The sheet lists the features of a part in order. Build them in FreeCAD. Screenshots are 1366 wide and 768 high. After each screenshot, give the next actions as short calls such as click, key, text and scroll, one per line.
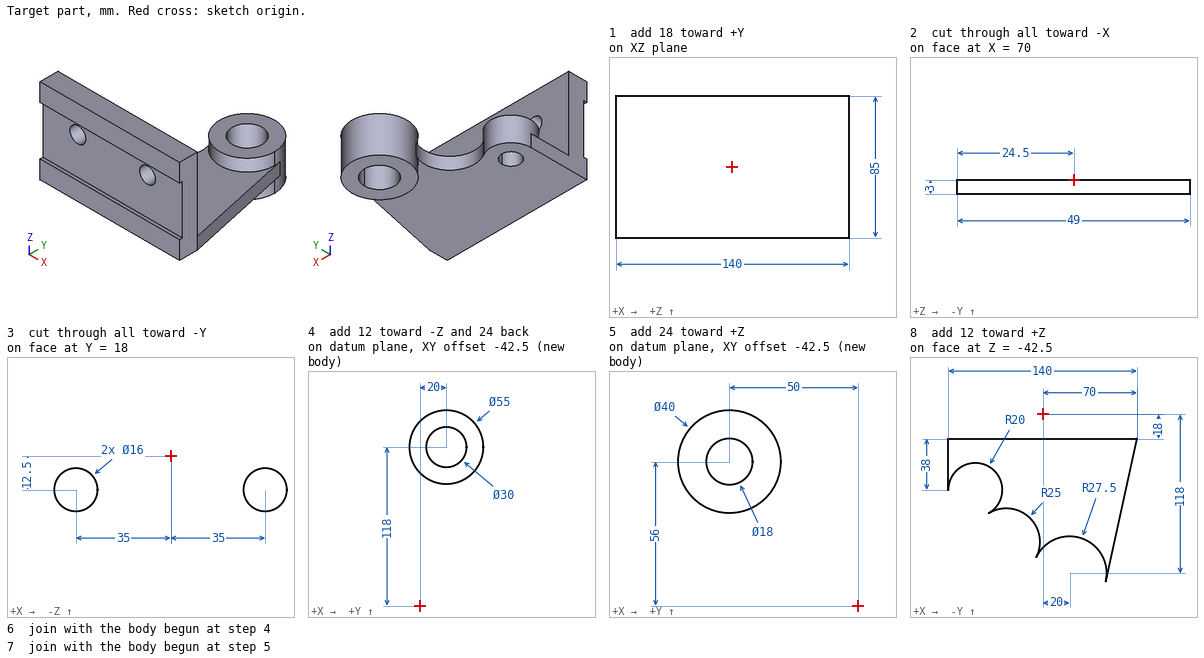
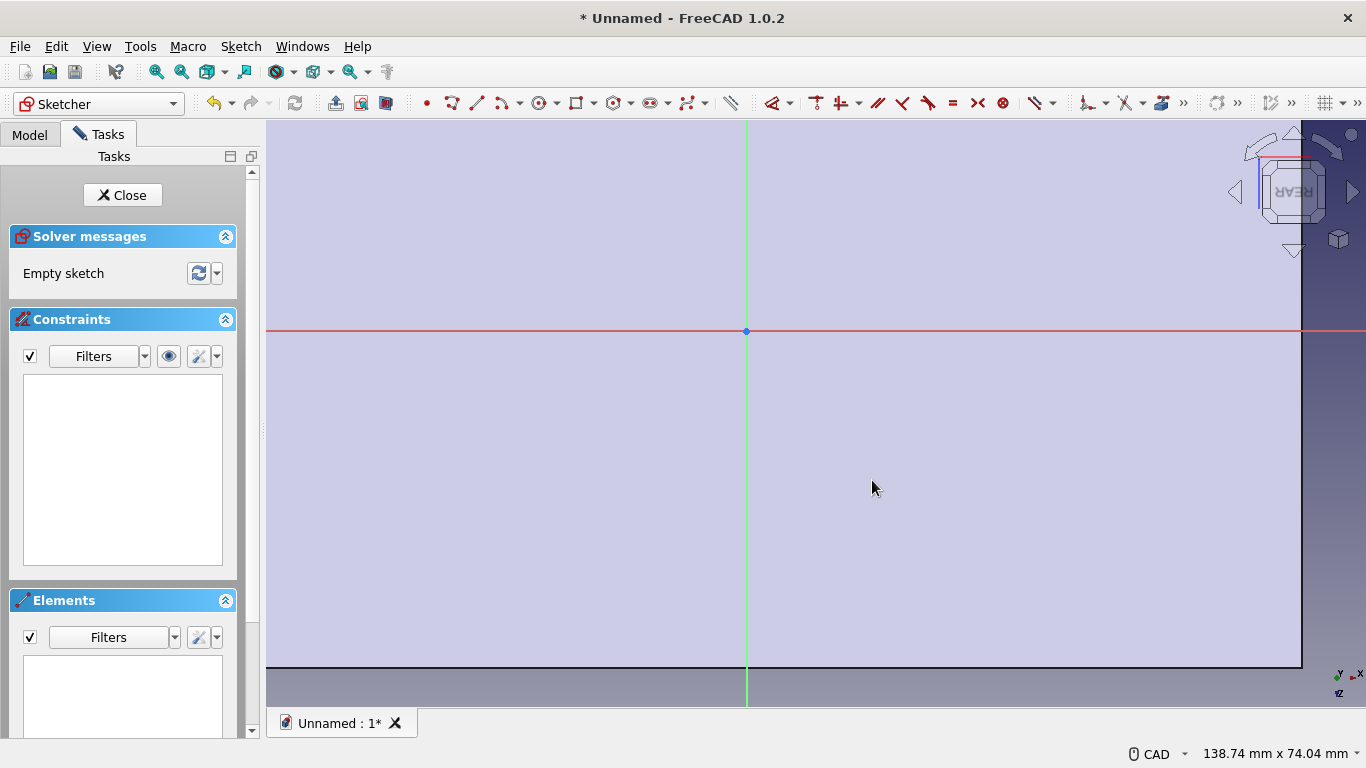
click(538, 104)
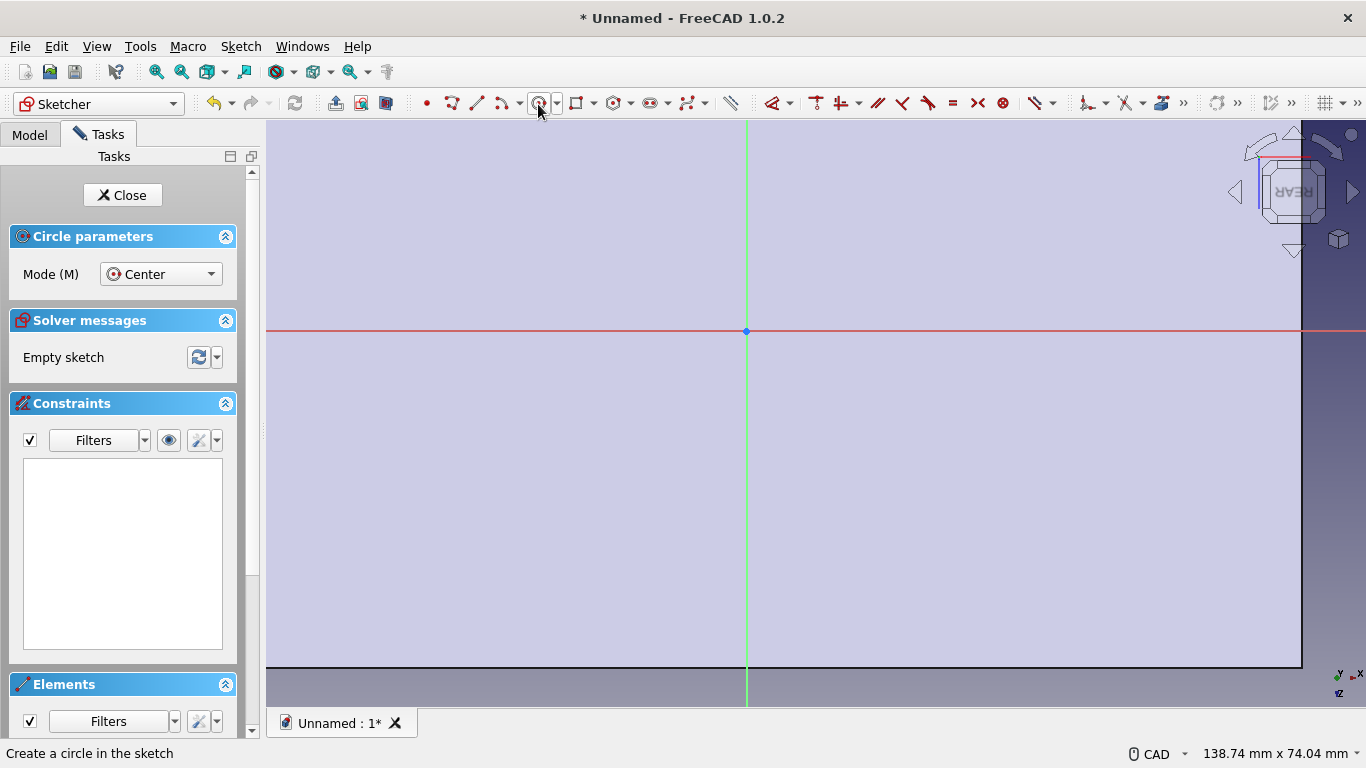
click(469, 430)
click(514, 386)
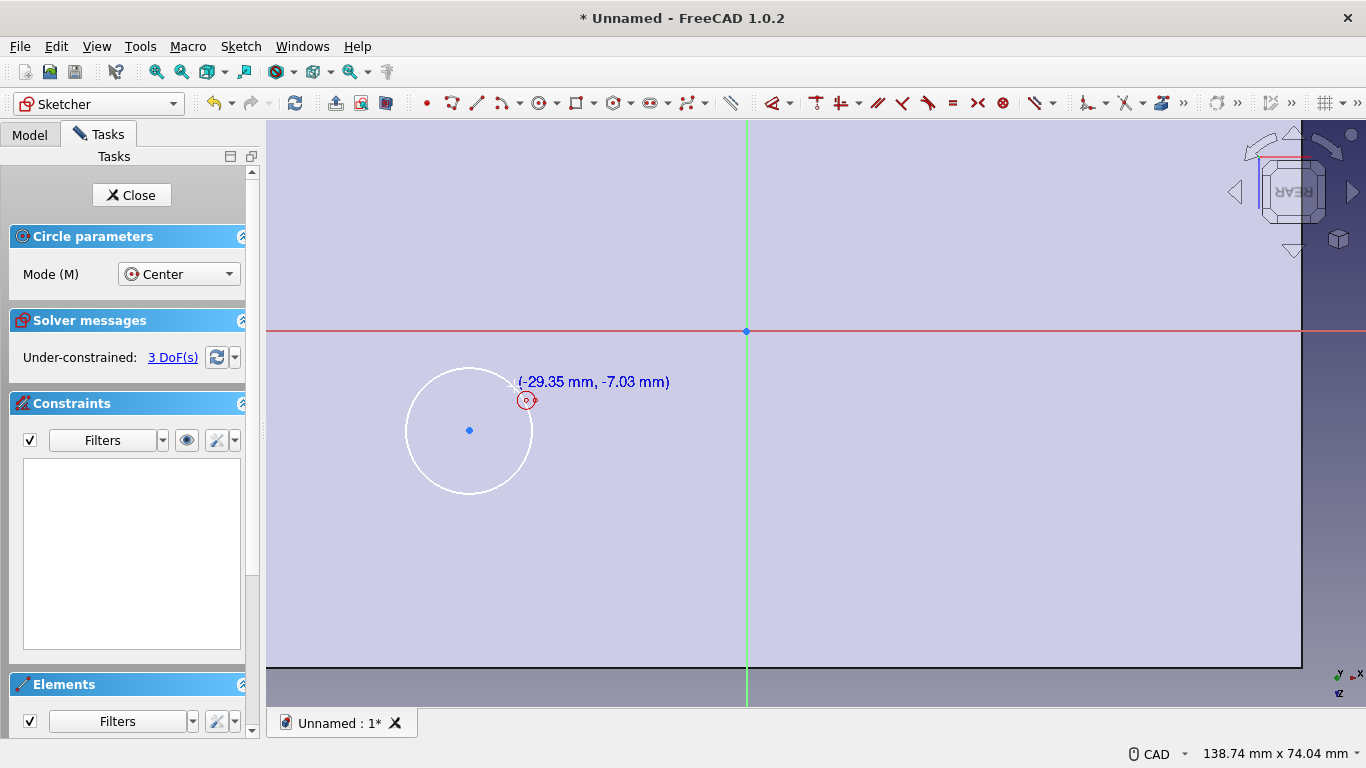
click(1024, 430)
click(1069, 386)
key(Escape)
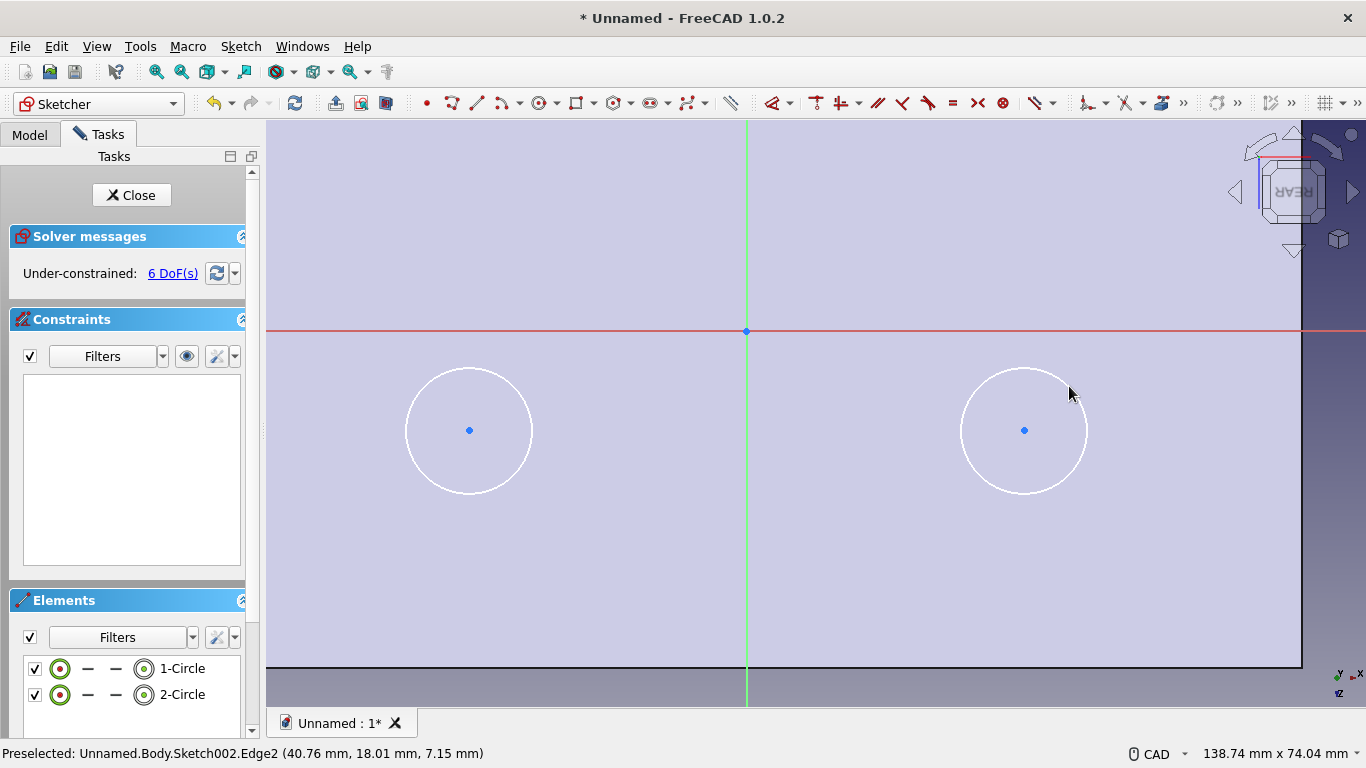
click(513, 386)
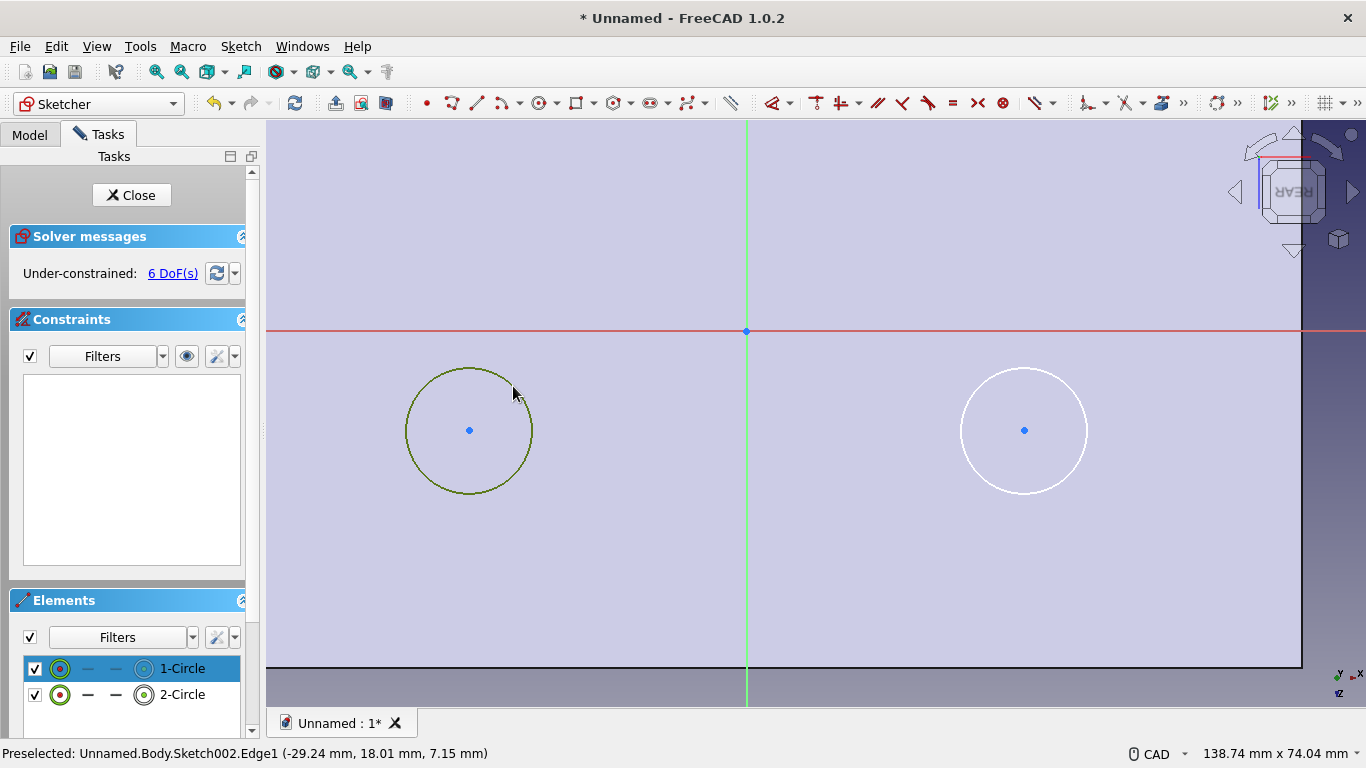
click(1068, 386)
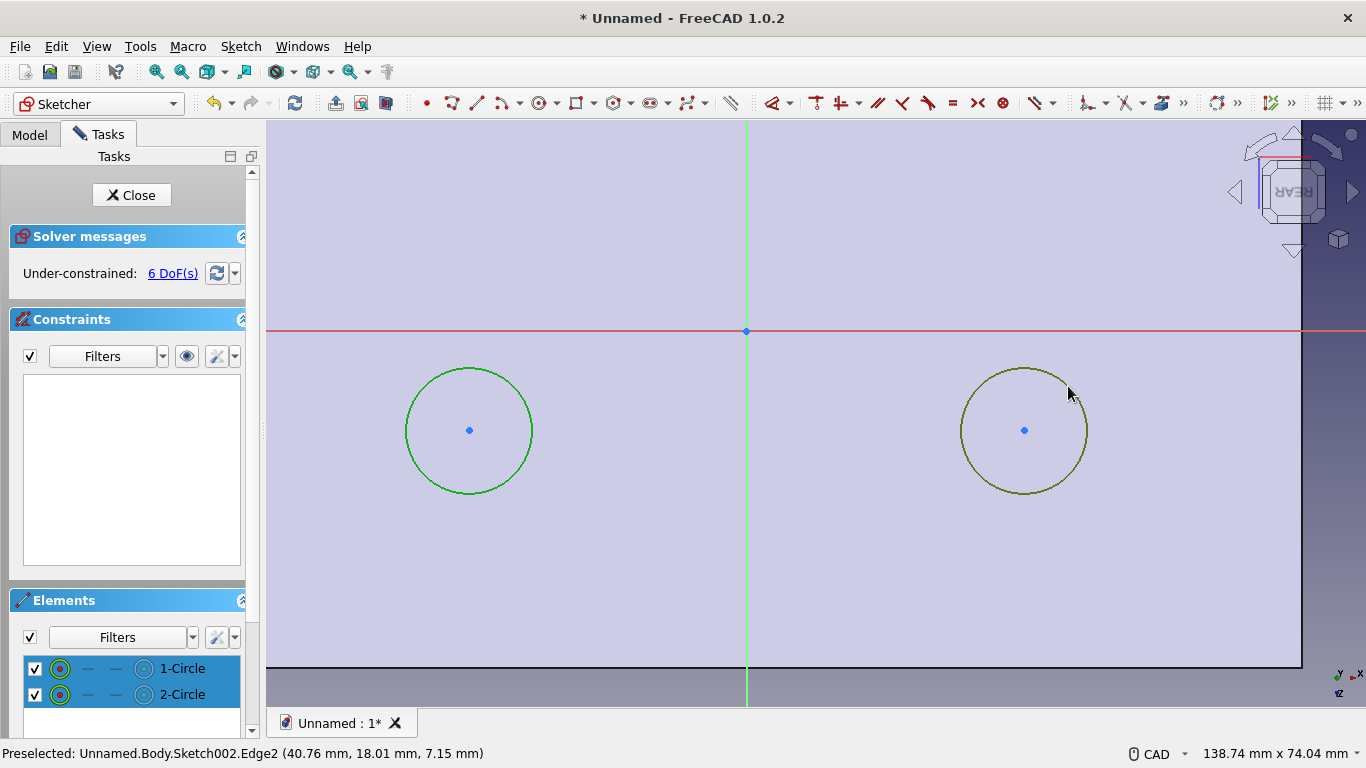
click(953, 104)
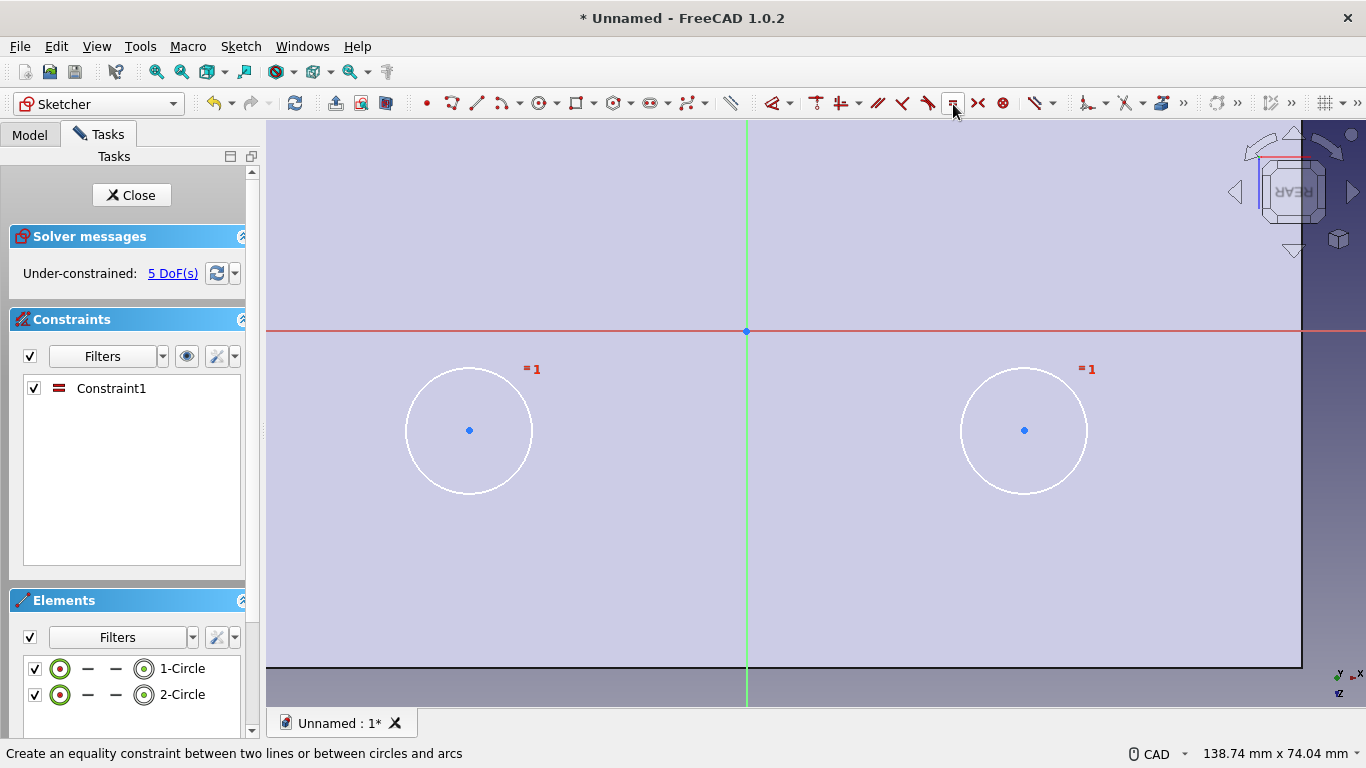
click(469, 431)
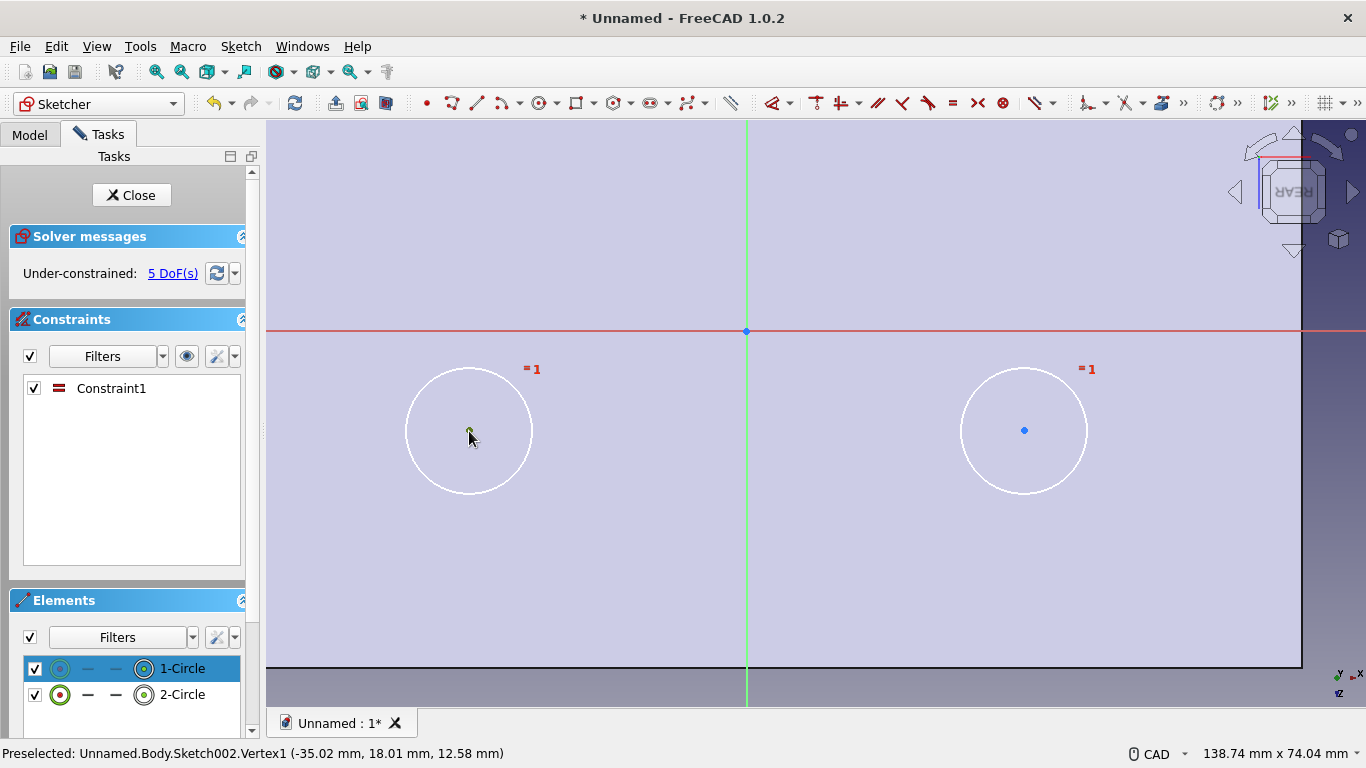
click(1024, 431)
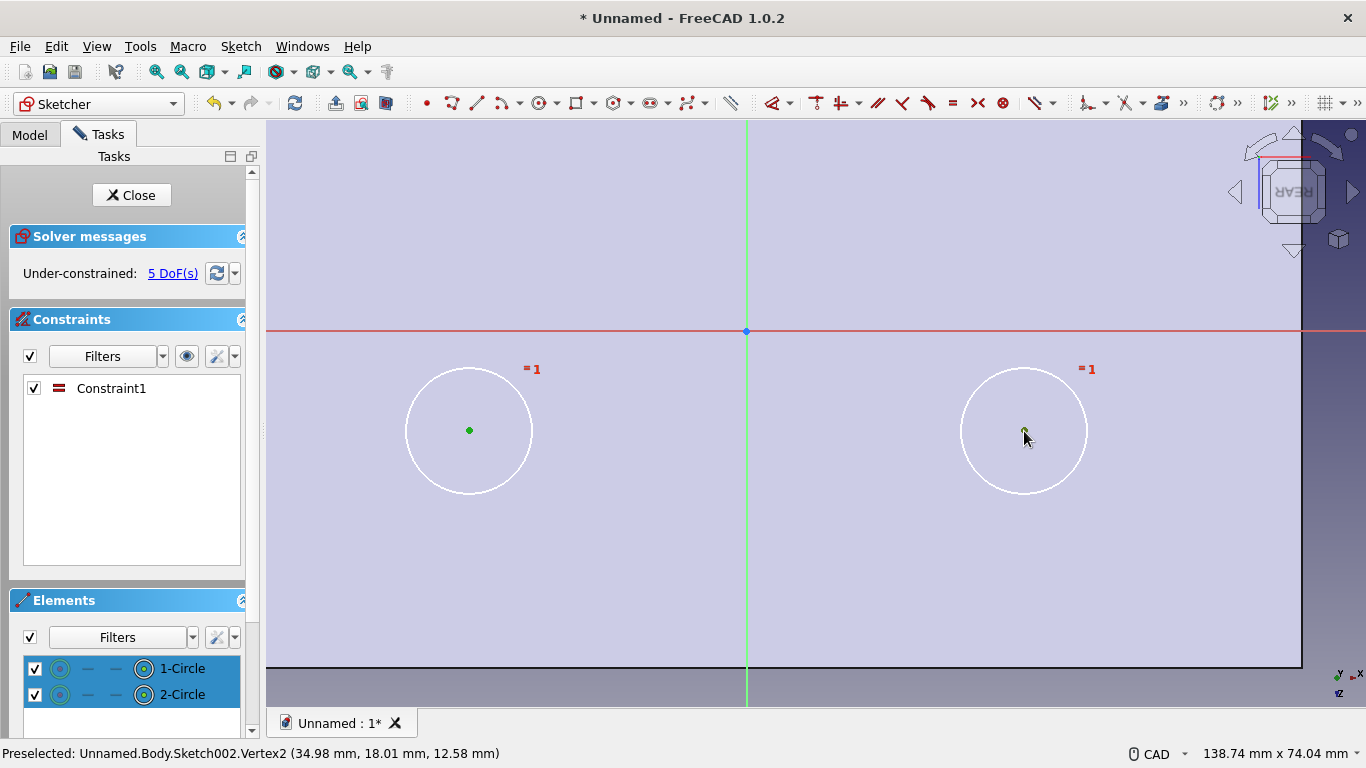
click(858, 104)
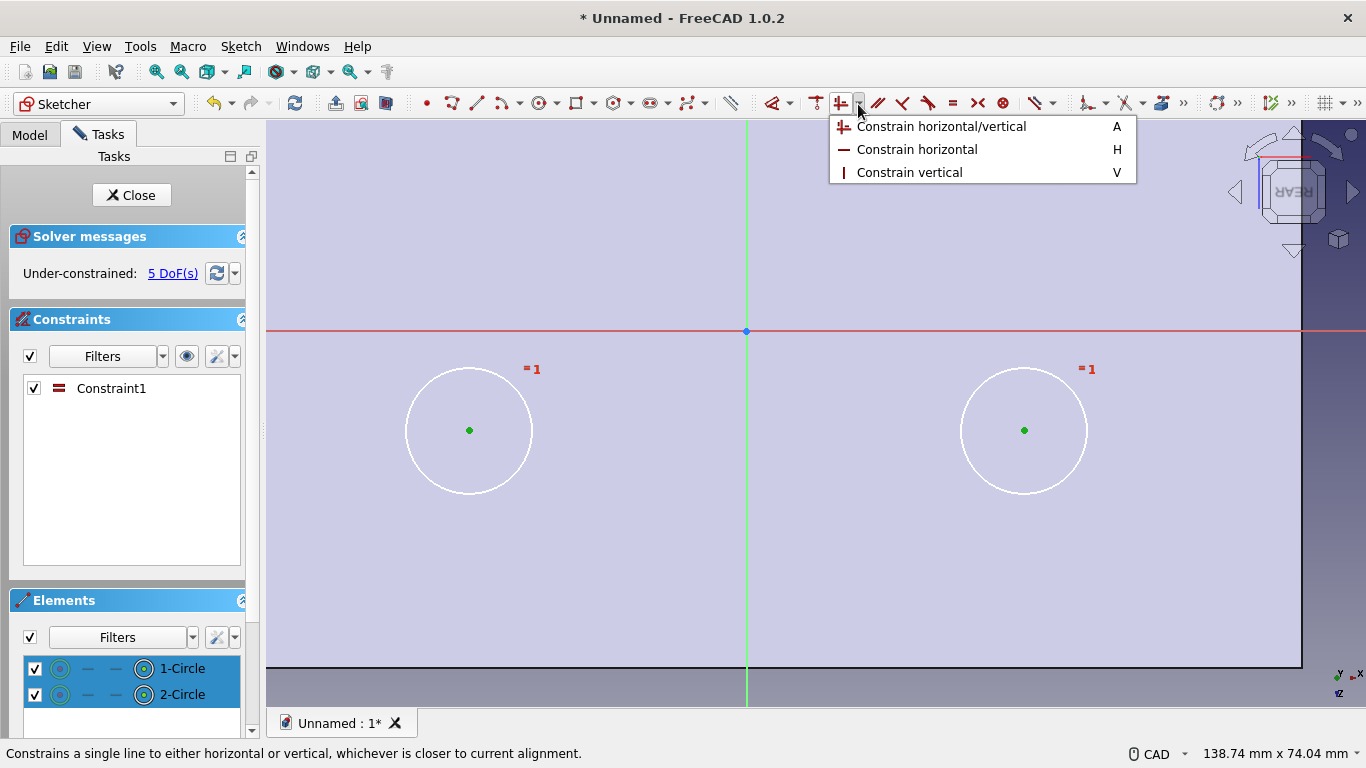
click(983, 150)